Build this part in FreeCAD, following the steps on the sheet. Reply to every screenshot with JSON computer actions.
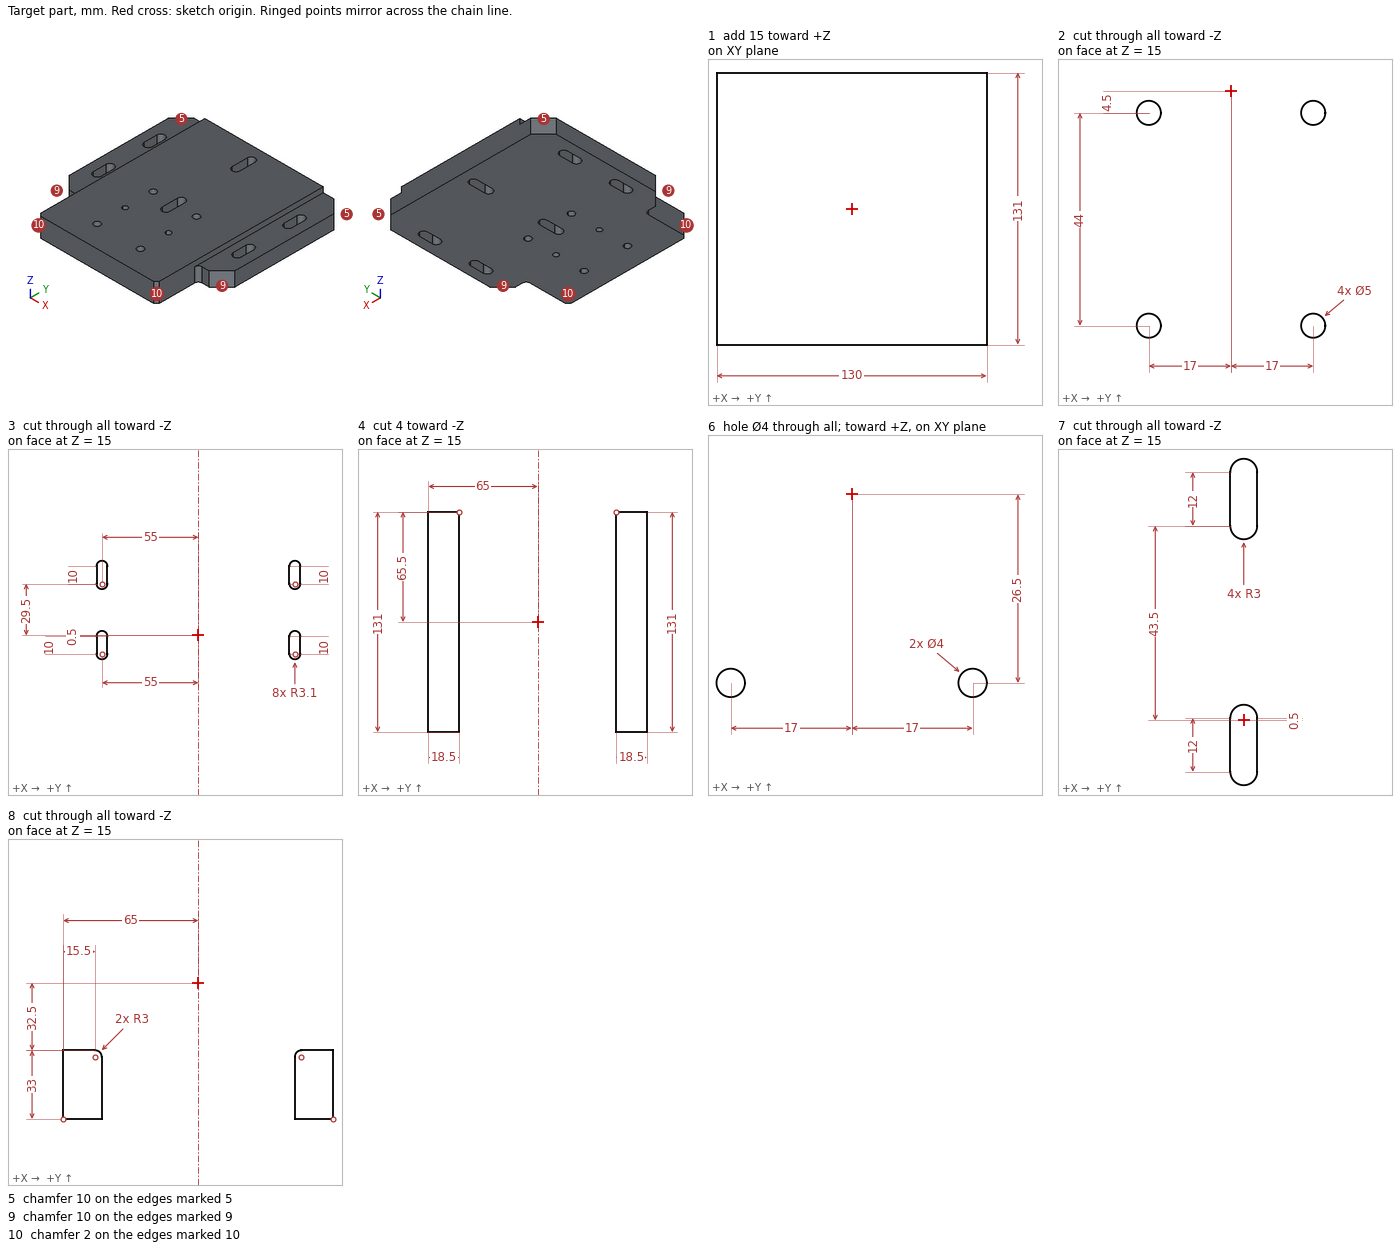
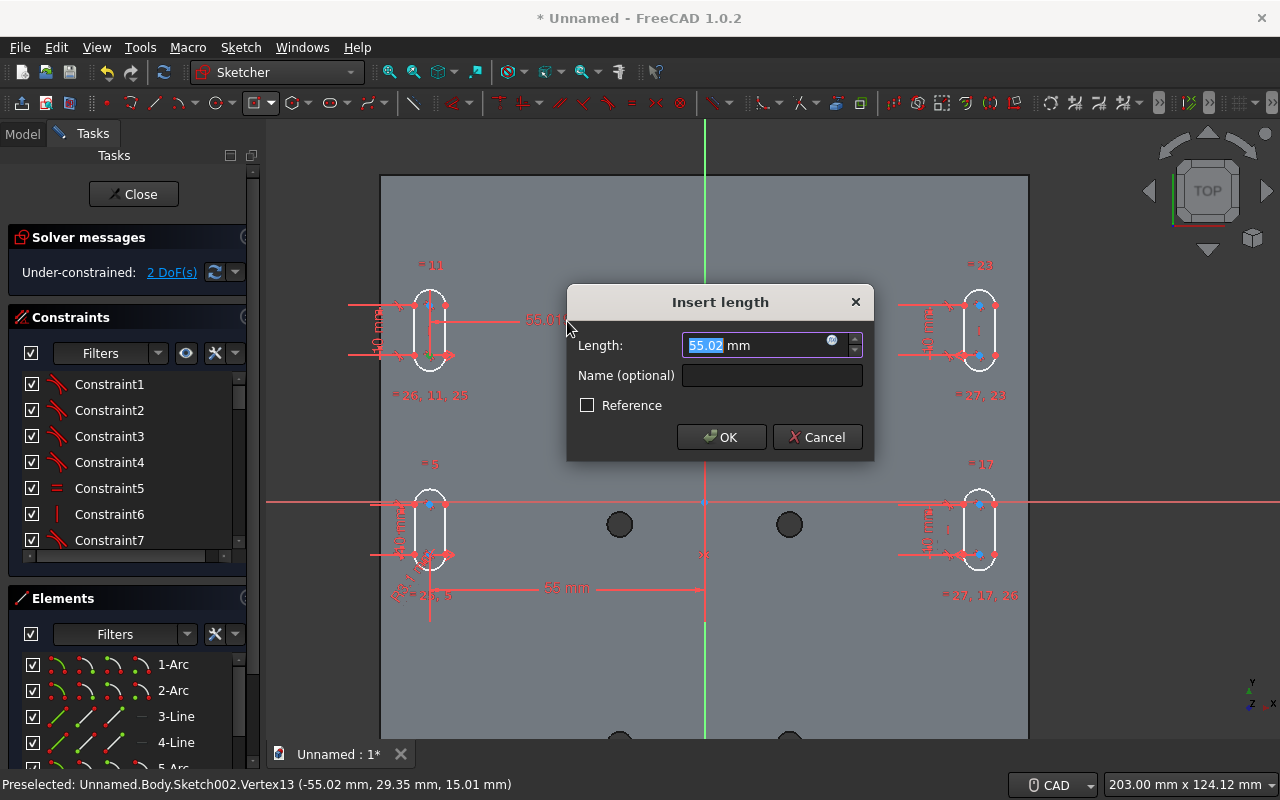
{"action": "type", "text": "55"}
{"action": "key", "text": "Return"}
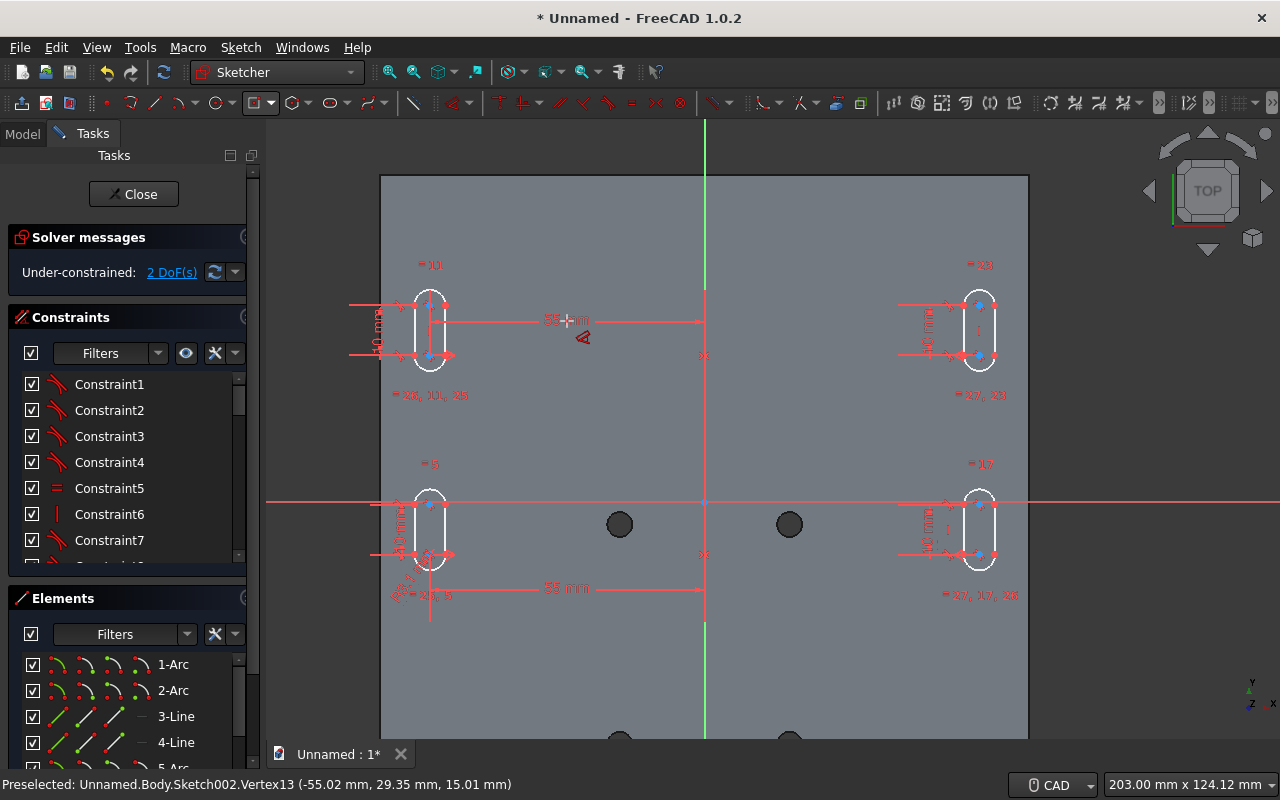
{"action": "scroll", "coordinate": [445, 505], "scroll_direction": "up", "scroll_amount": 14}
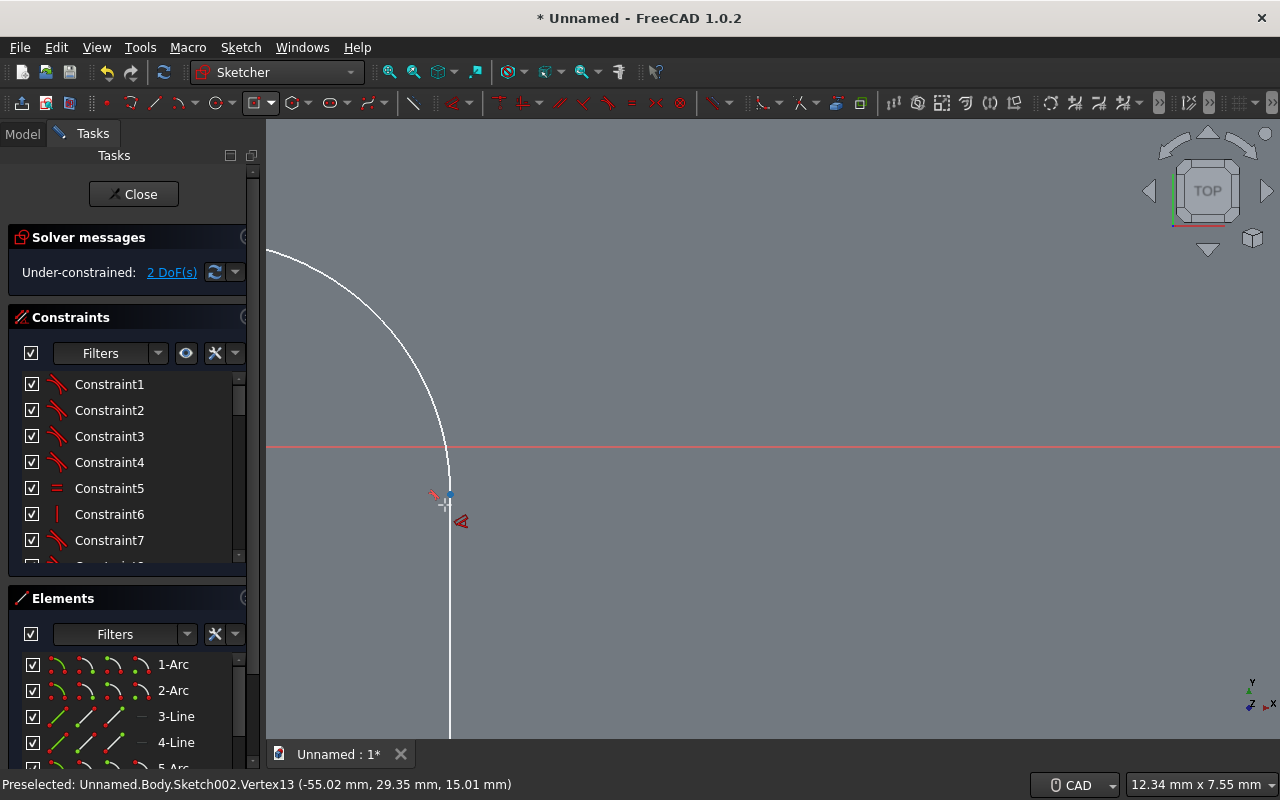
{"action": "left_click", "coordinate": [450, 494]}
{"action": "left_click", "coordinate": [416, 470]}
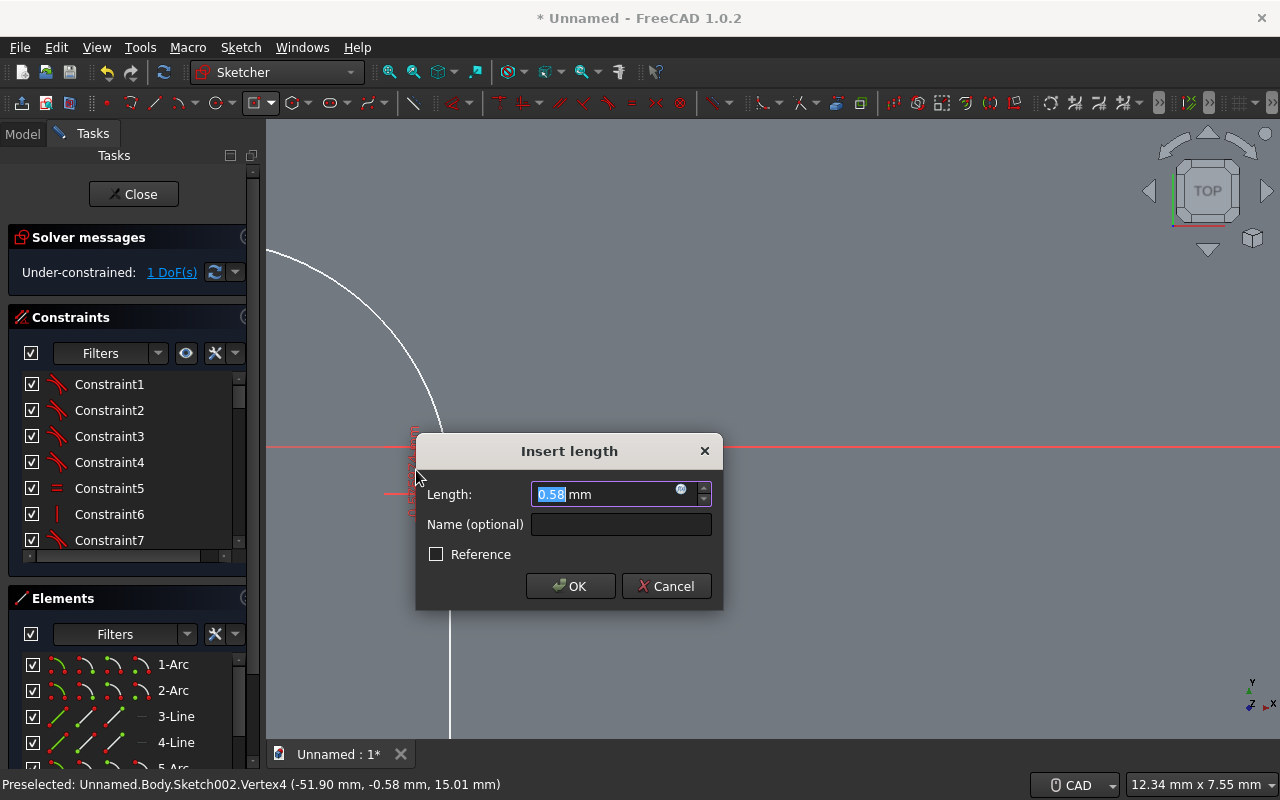
{"action": "type", "text": "0.5"}
{"action": "key", "text": "Return"}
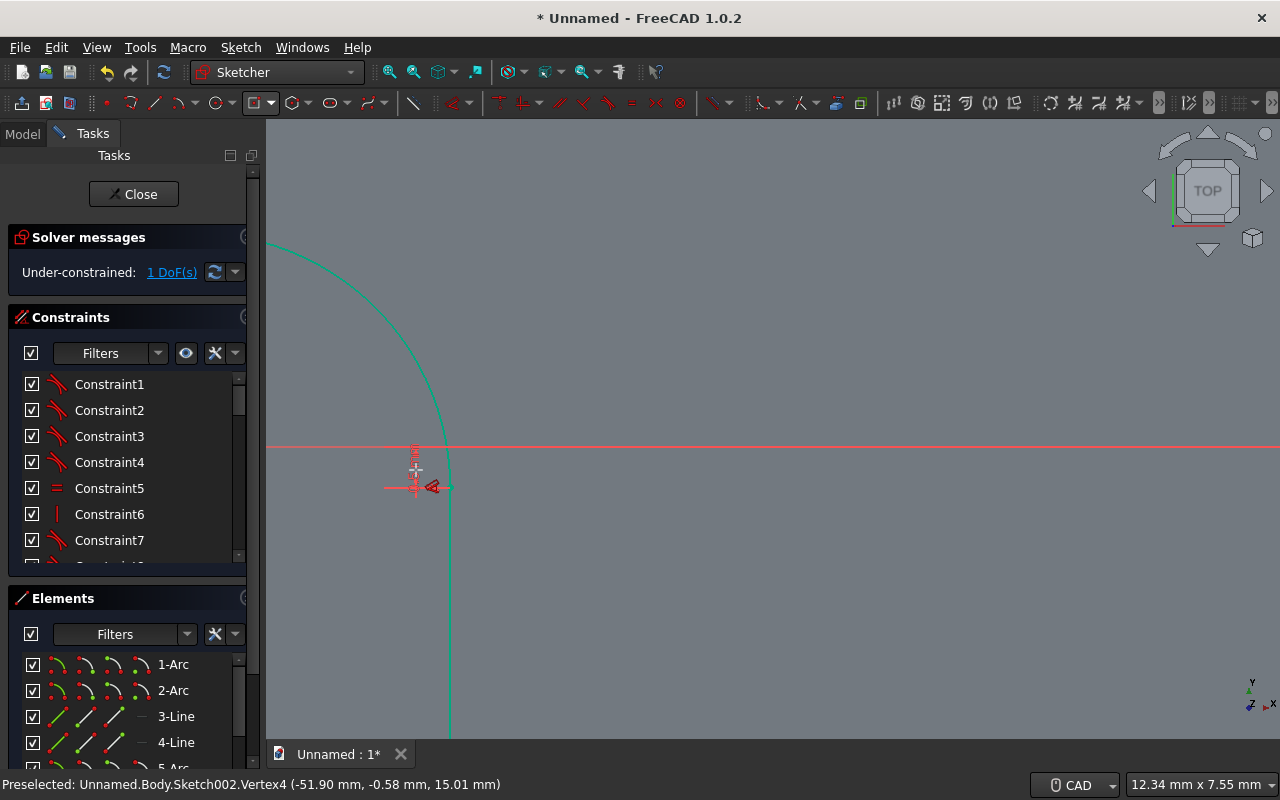
{"action": "scroll", "coordinate": [445, 505], "scroll_direction": "down", "scroll_amount": 14}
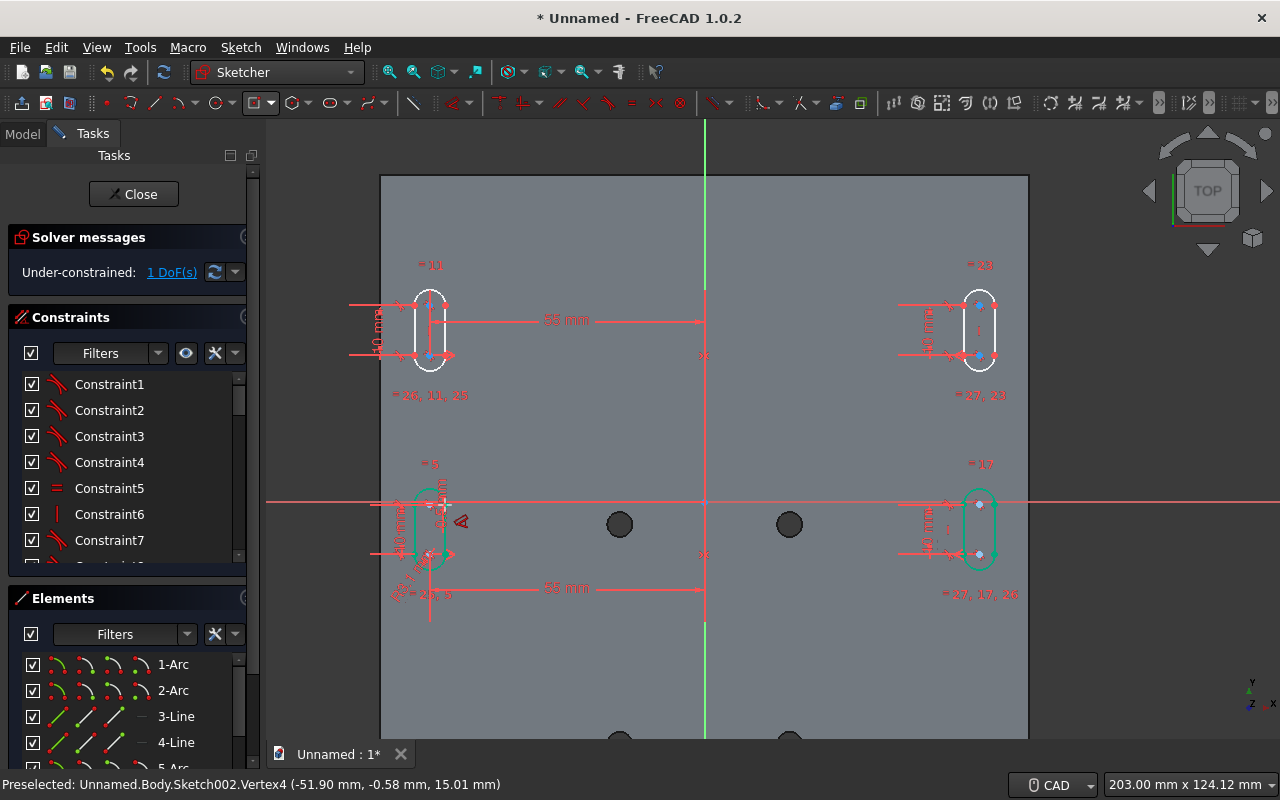
{"action": "left_click", "coordinate": [415, 355]}
{"action": "left_click", "coordinate": [381, 429]}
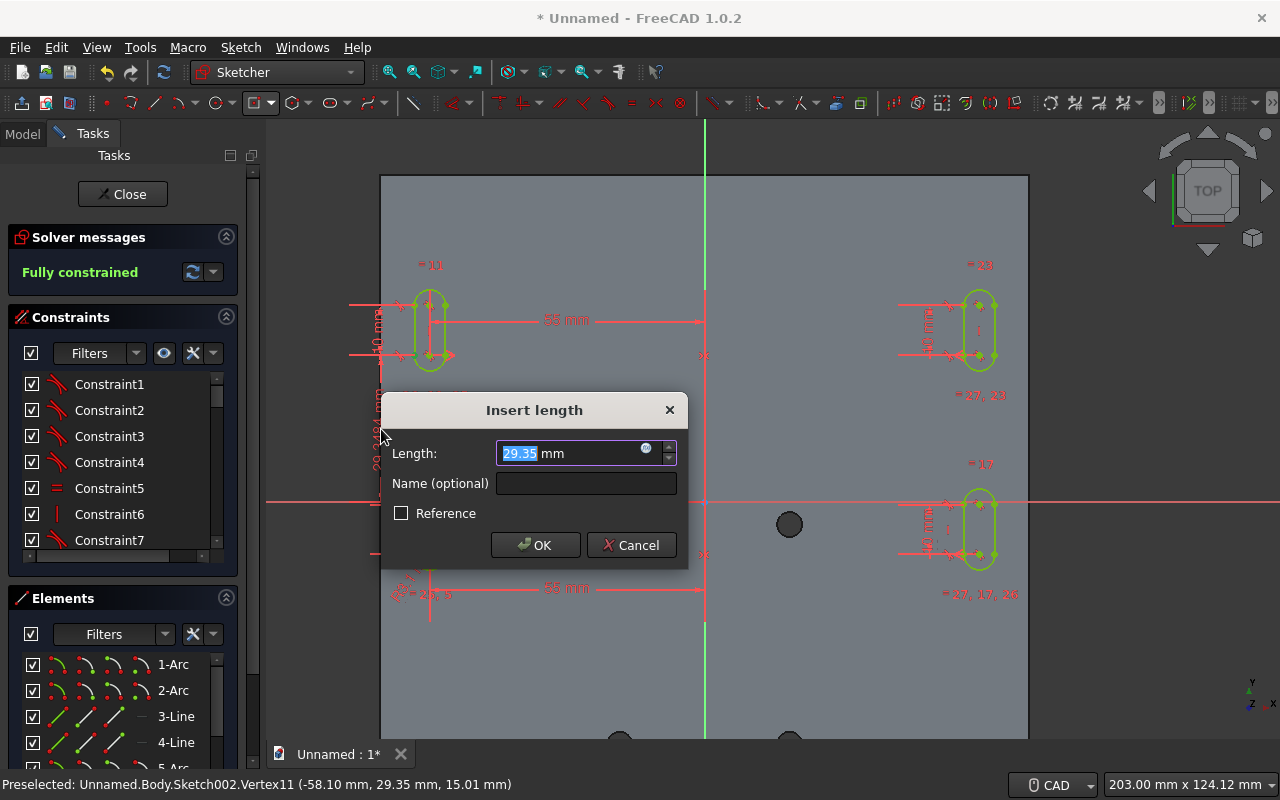
{"action": "type", "text": "29.5"}
{"action": "key", "text": "Return"}
{"action": "key", "text": "Escape"}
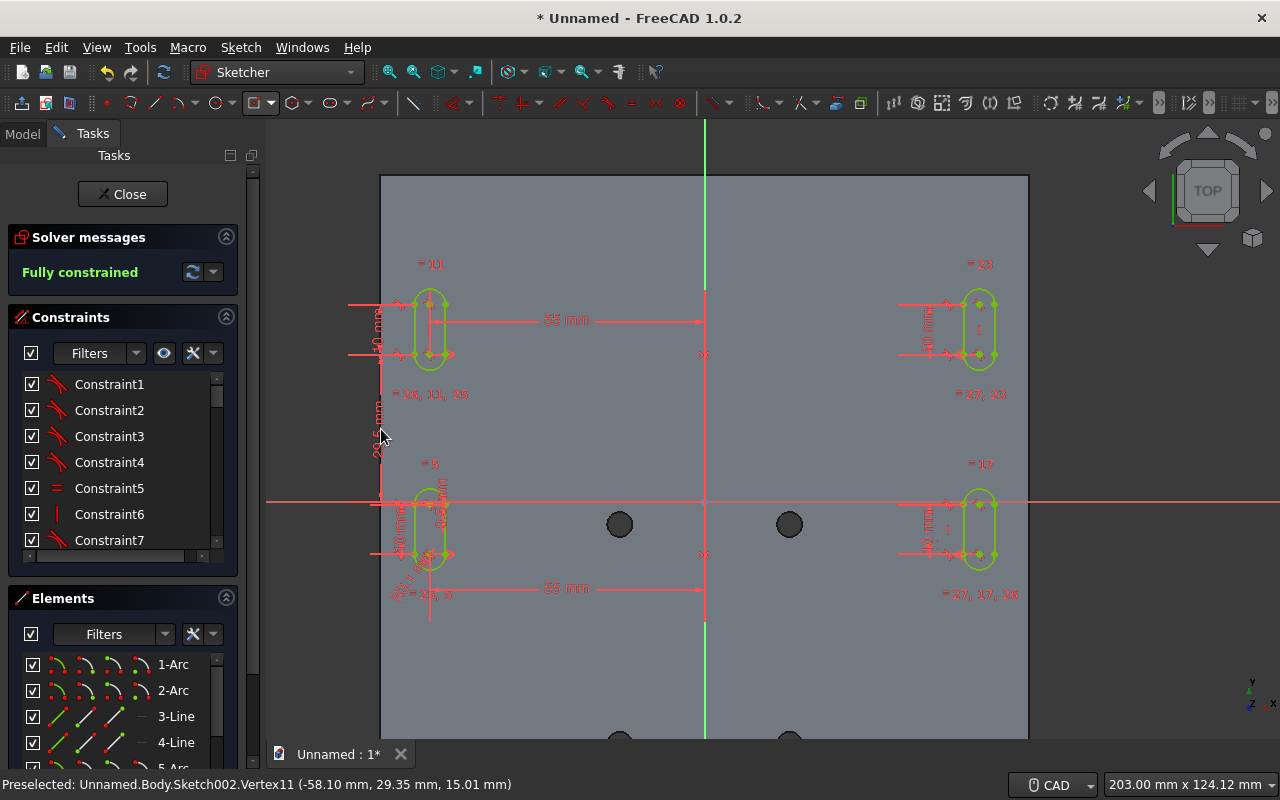
{"action": "left_click", "coordinate": [123, 194]}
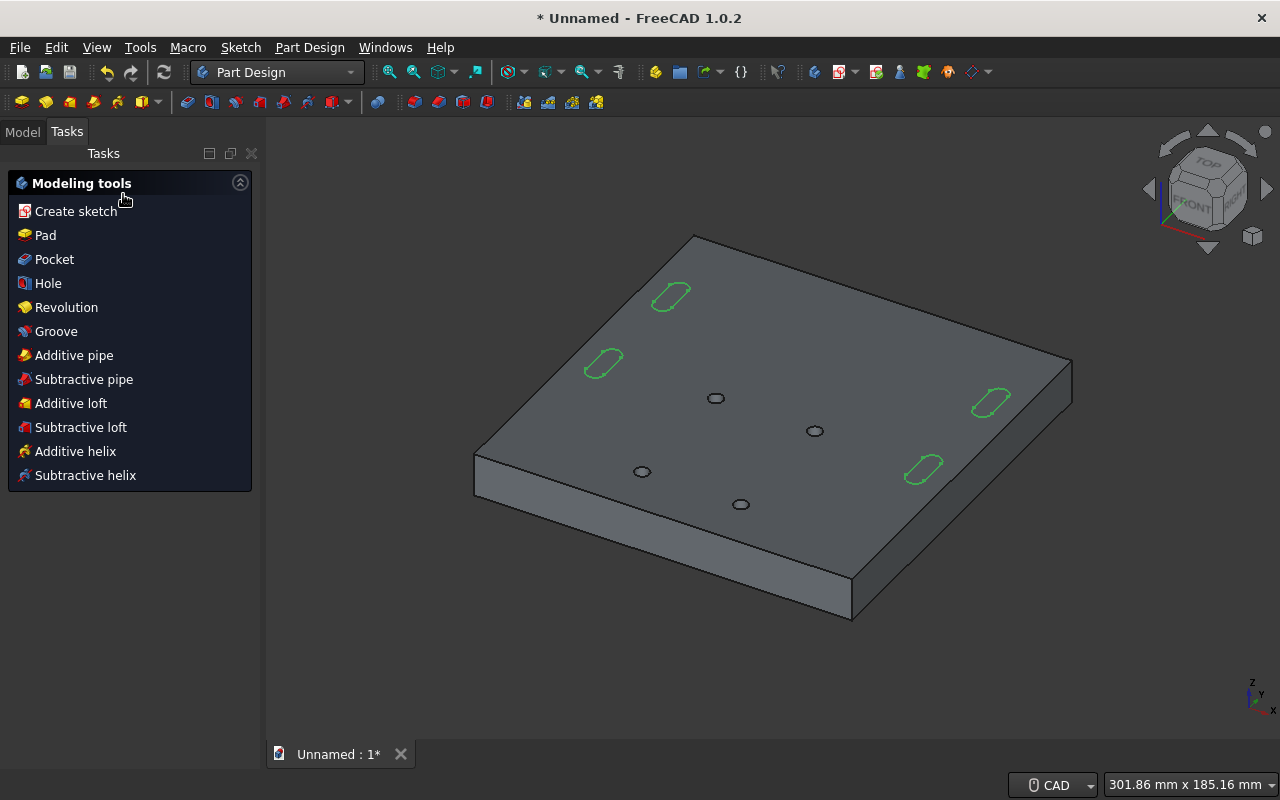
{"action": "left_click", "coordinate": [188, 102]}